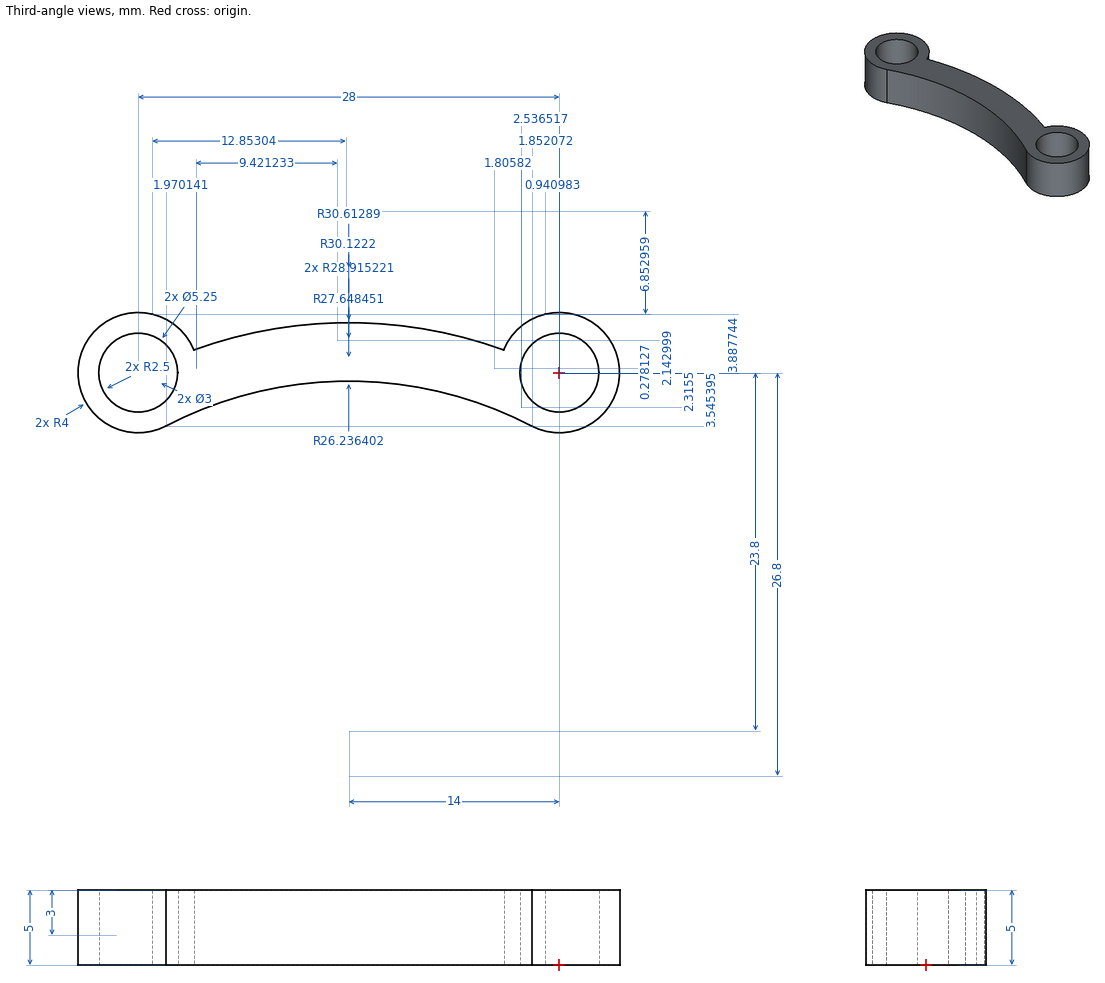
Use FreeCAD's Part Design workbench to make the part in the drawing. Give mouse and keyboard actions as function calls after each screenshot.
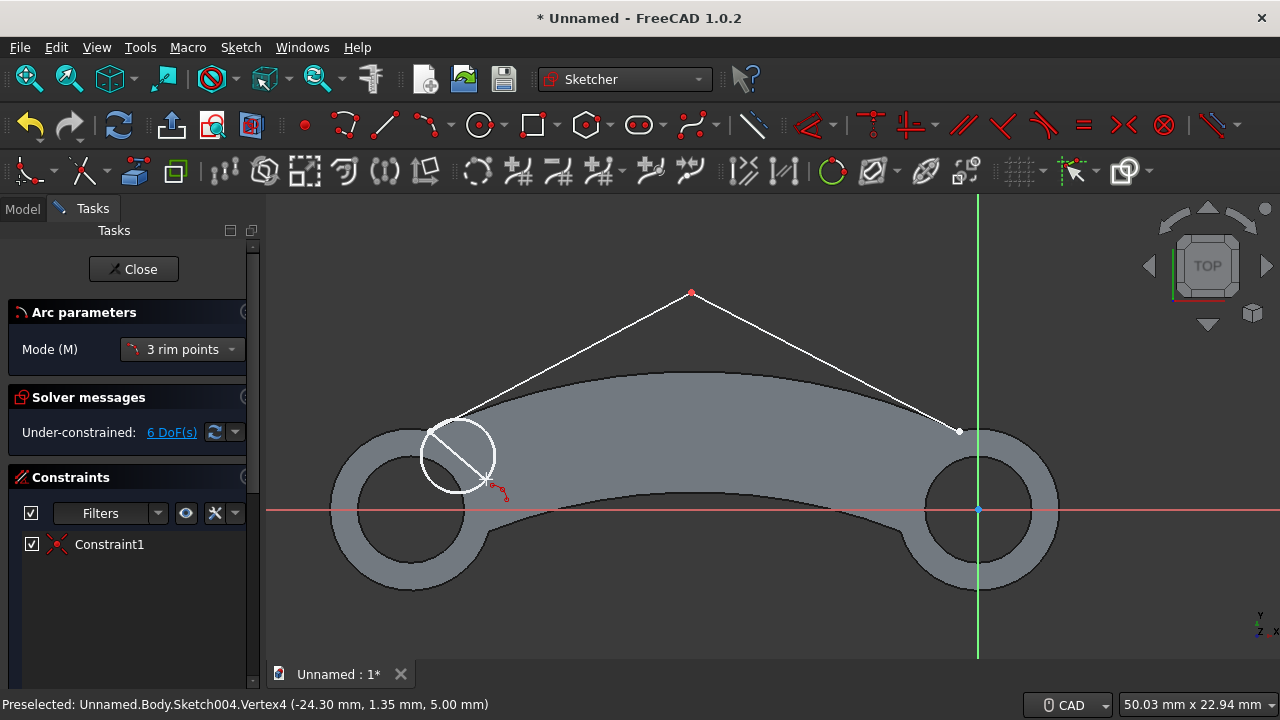
scroll(464, 448, up, 3)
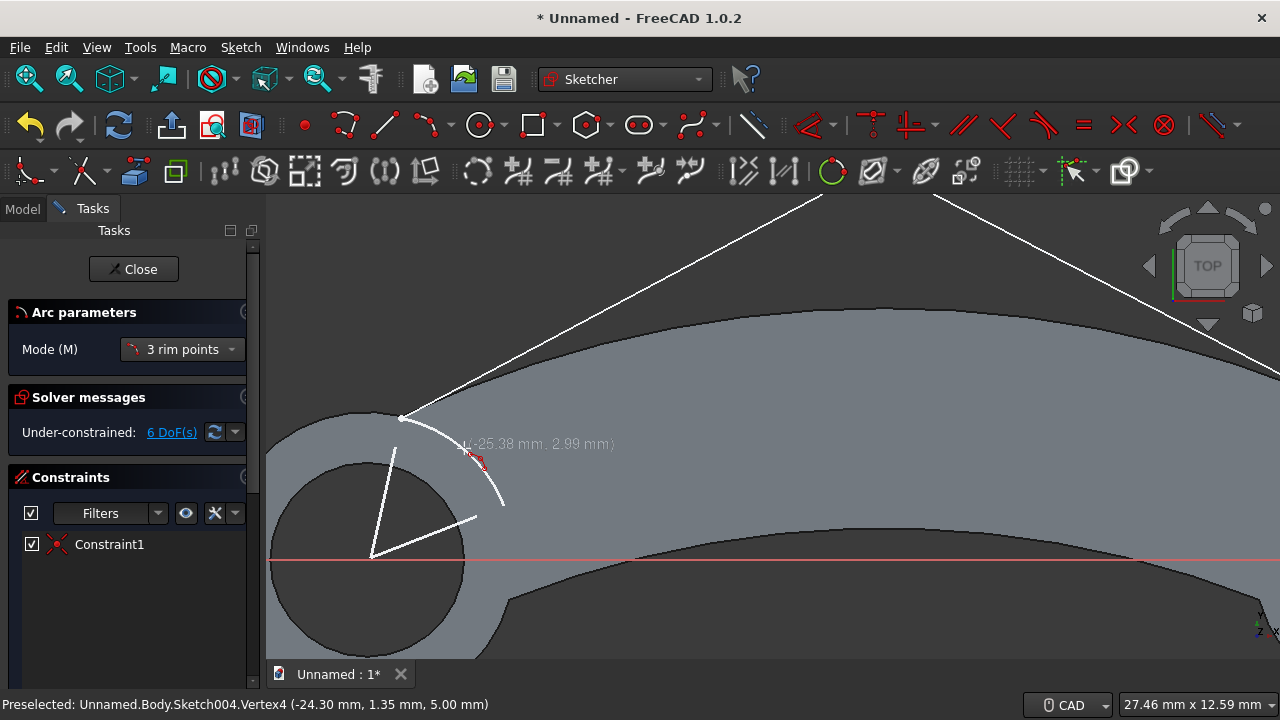
click(464, 448)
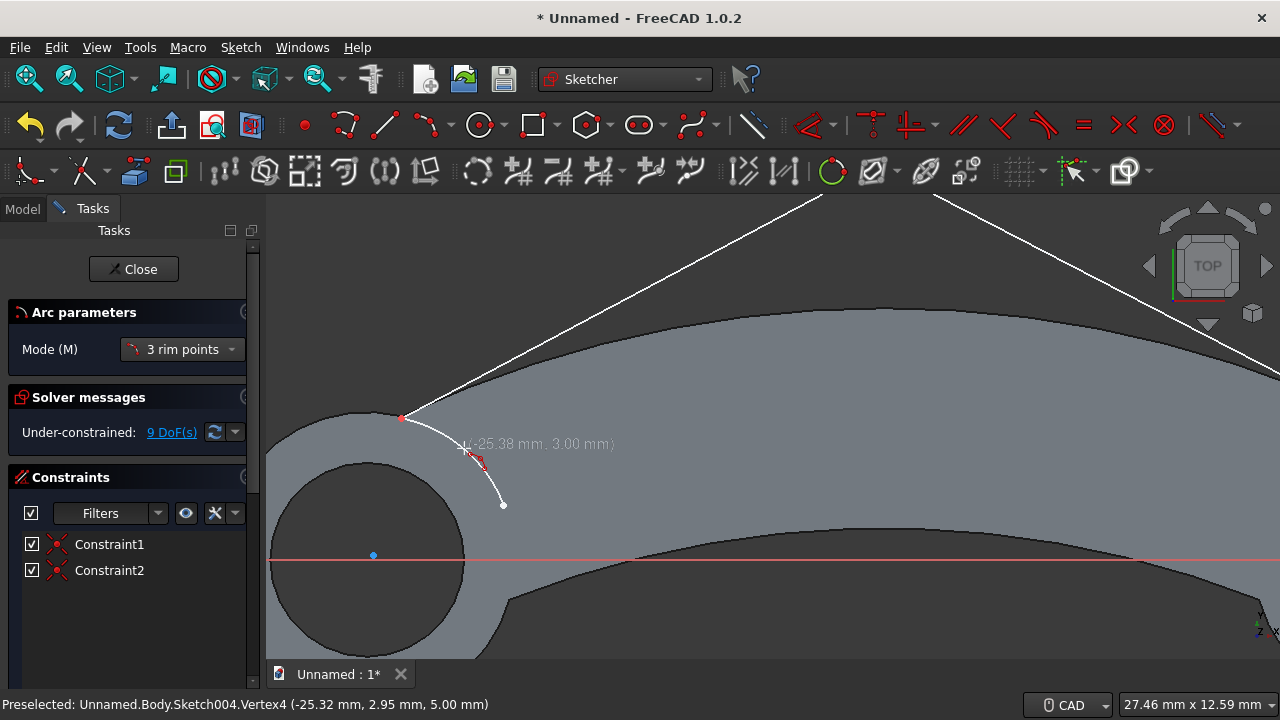
click(504, 506)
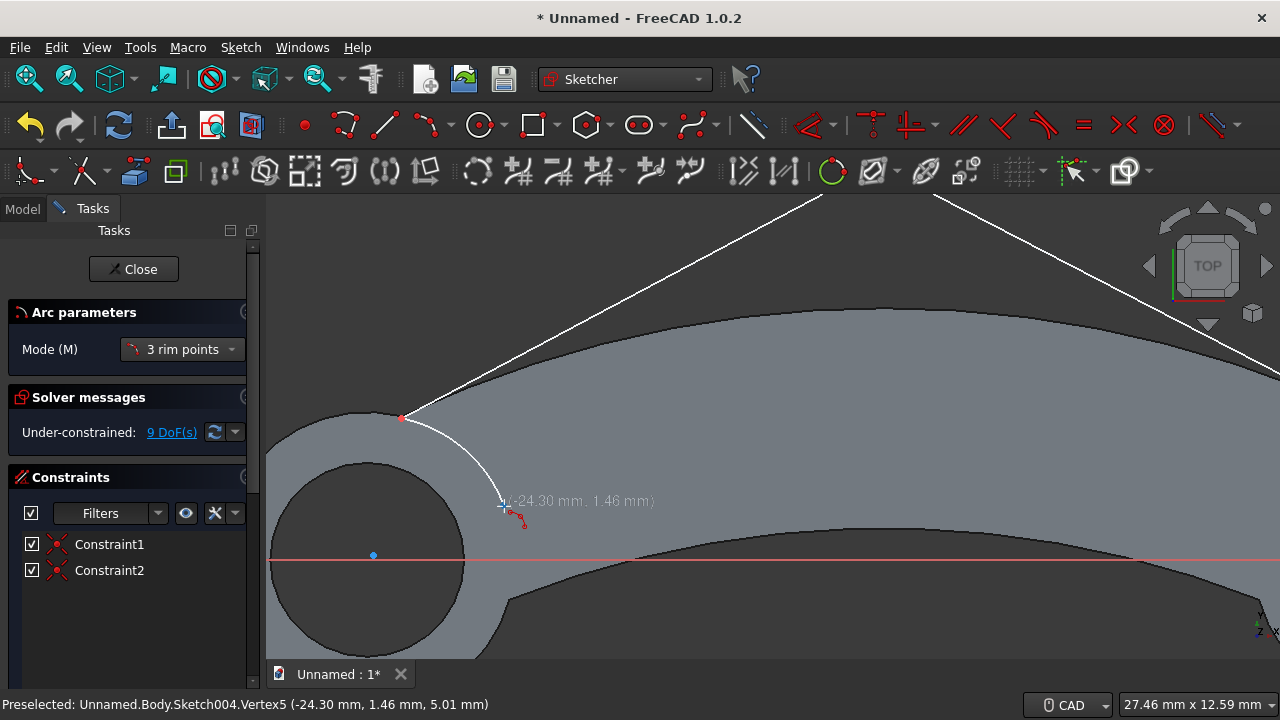
scroll(465, 506, down, 3)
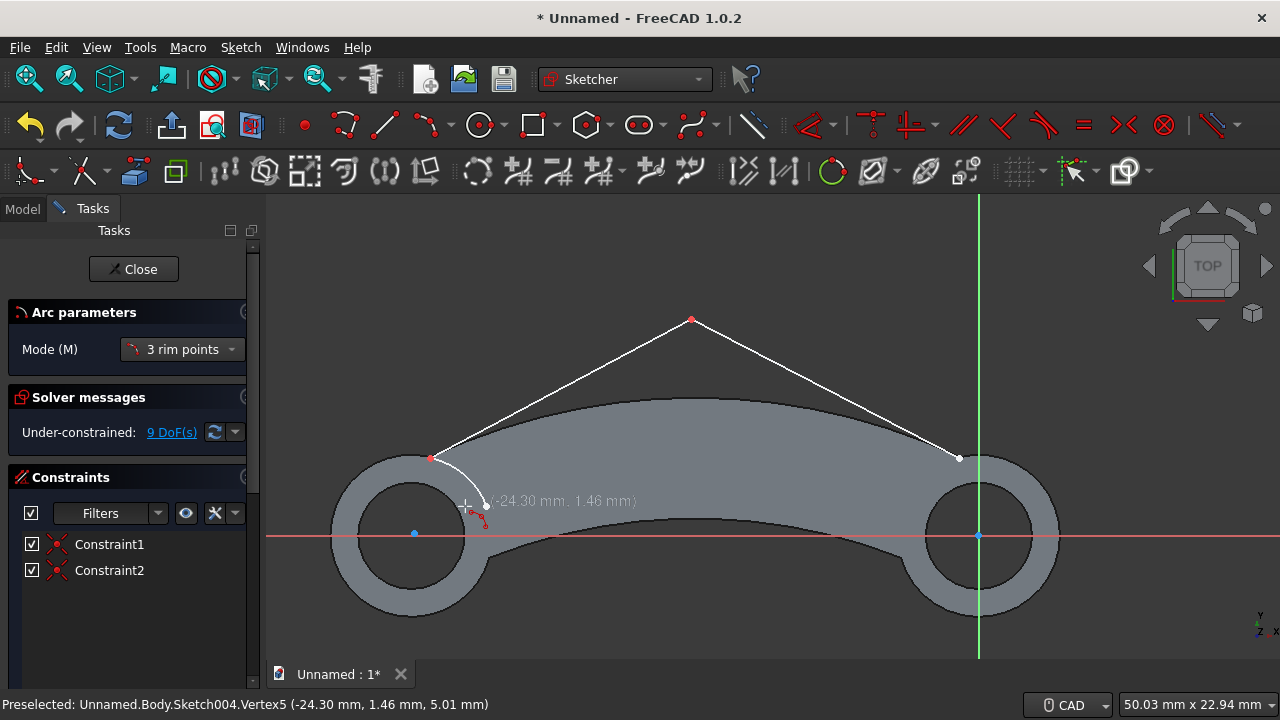
click(904, 505)
click(695, 469)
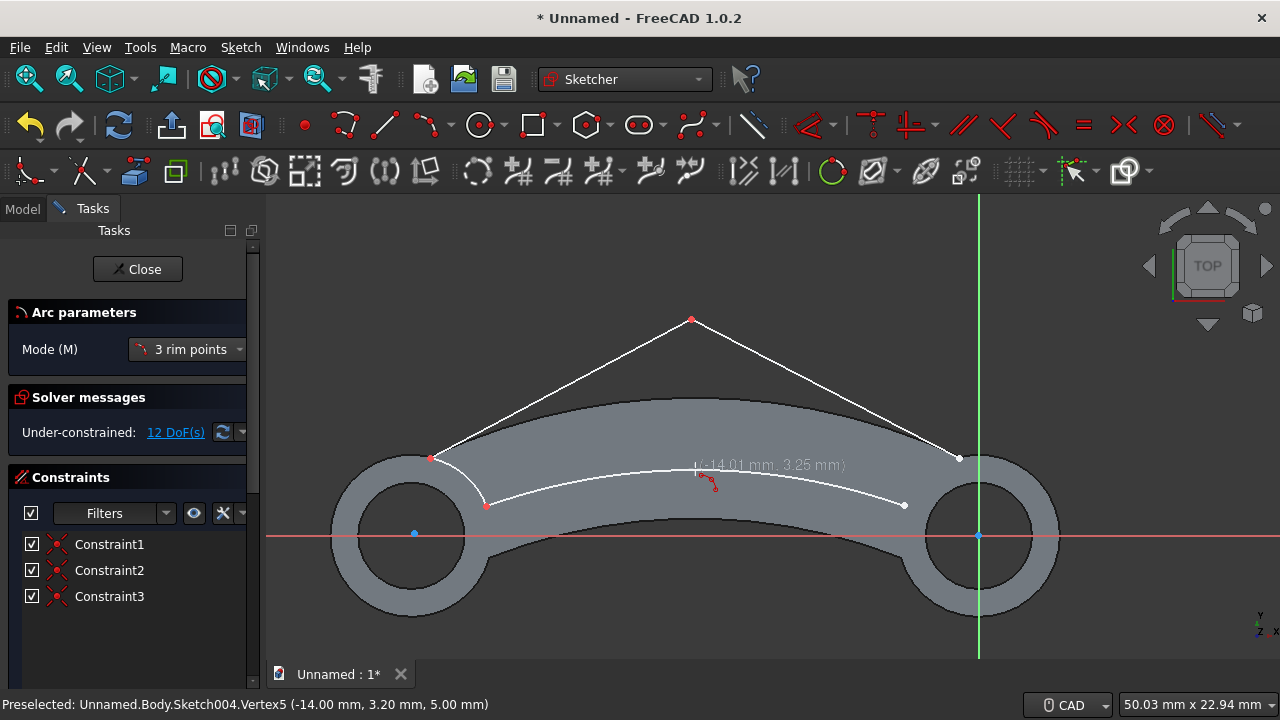
click(904, 506)
click(959, 458)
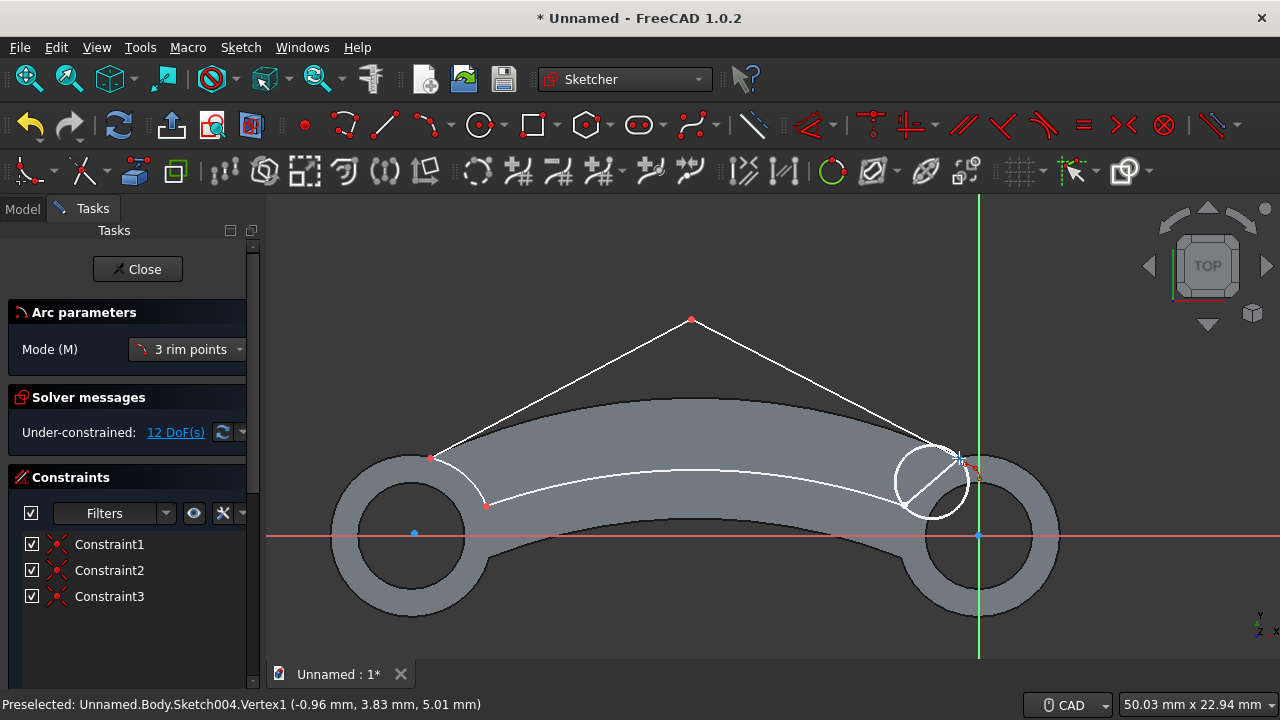
scroll(926, 474, up, 3)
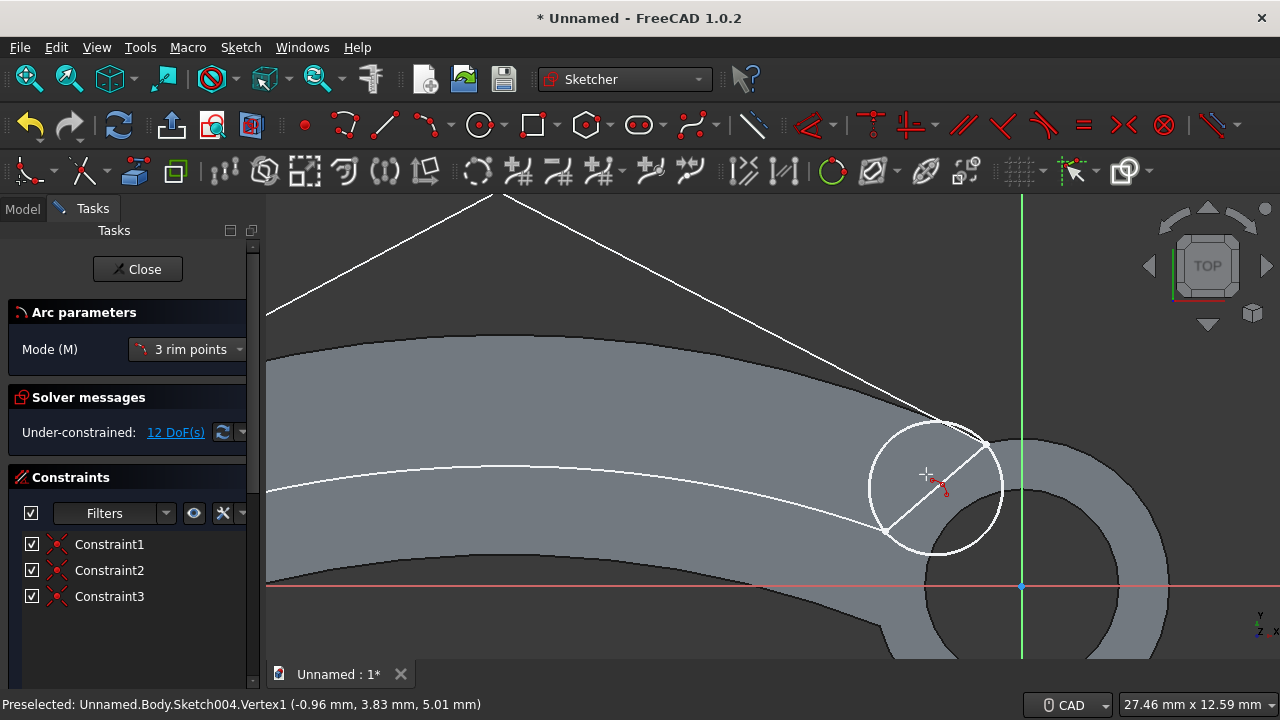
click(925, 474)
key(Escape)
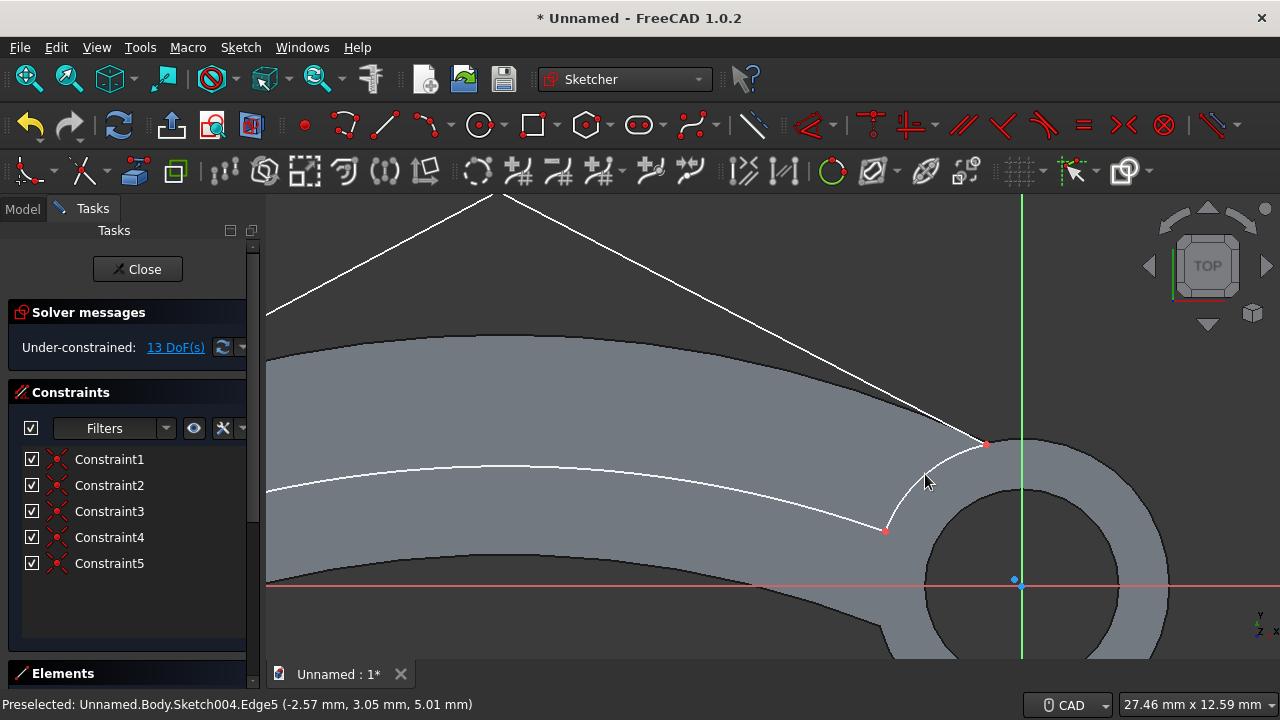
drag(1005, 570, 1032, 596)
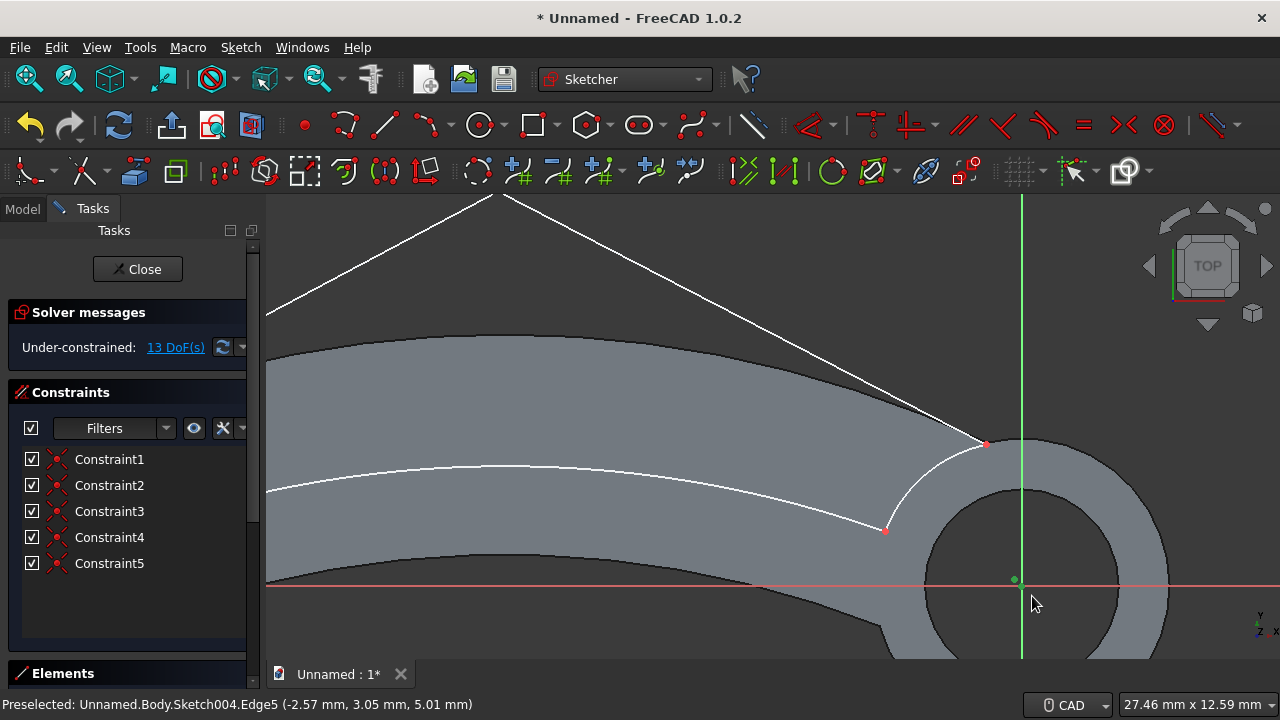
click(872, 126)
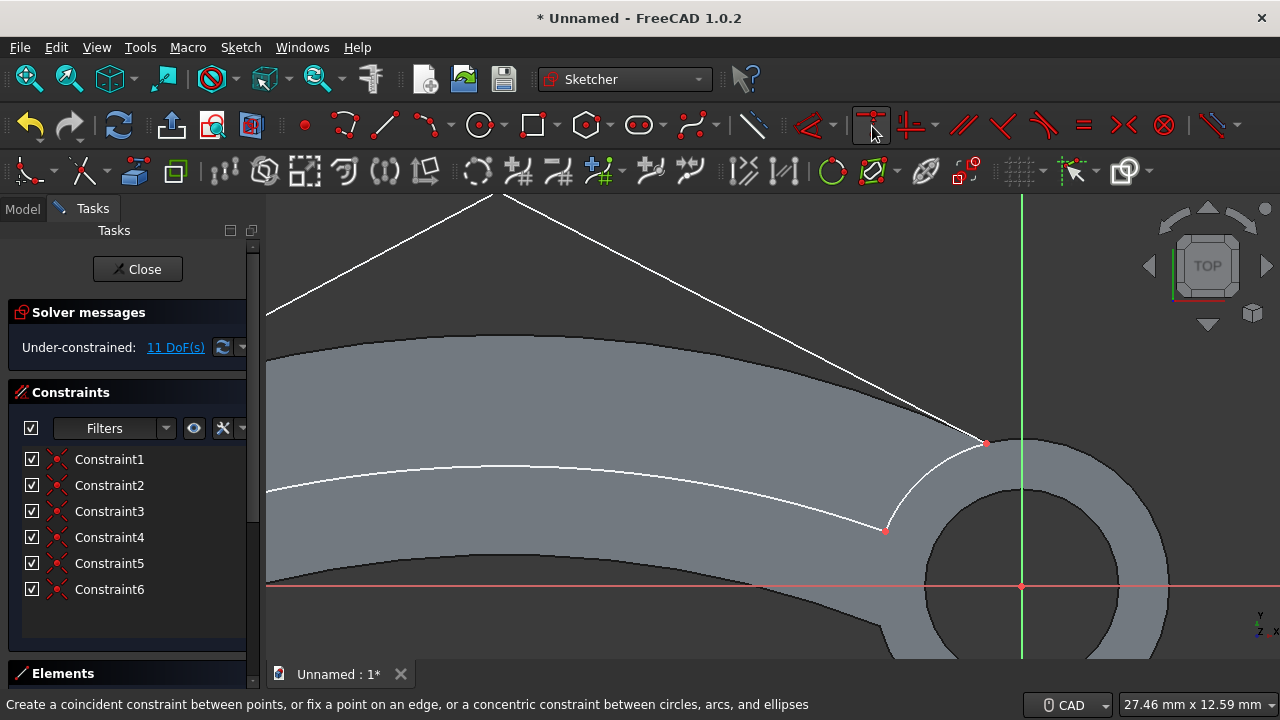
scroll(926, 473, down, 3)